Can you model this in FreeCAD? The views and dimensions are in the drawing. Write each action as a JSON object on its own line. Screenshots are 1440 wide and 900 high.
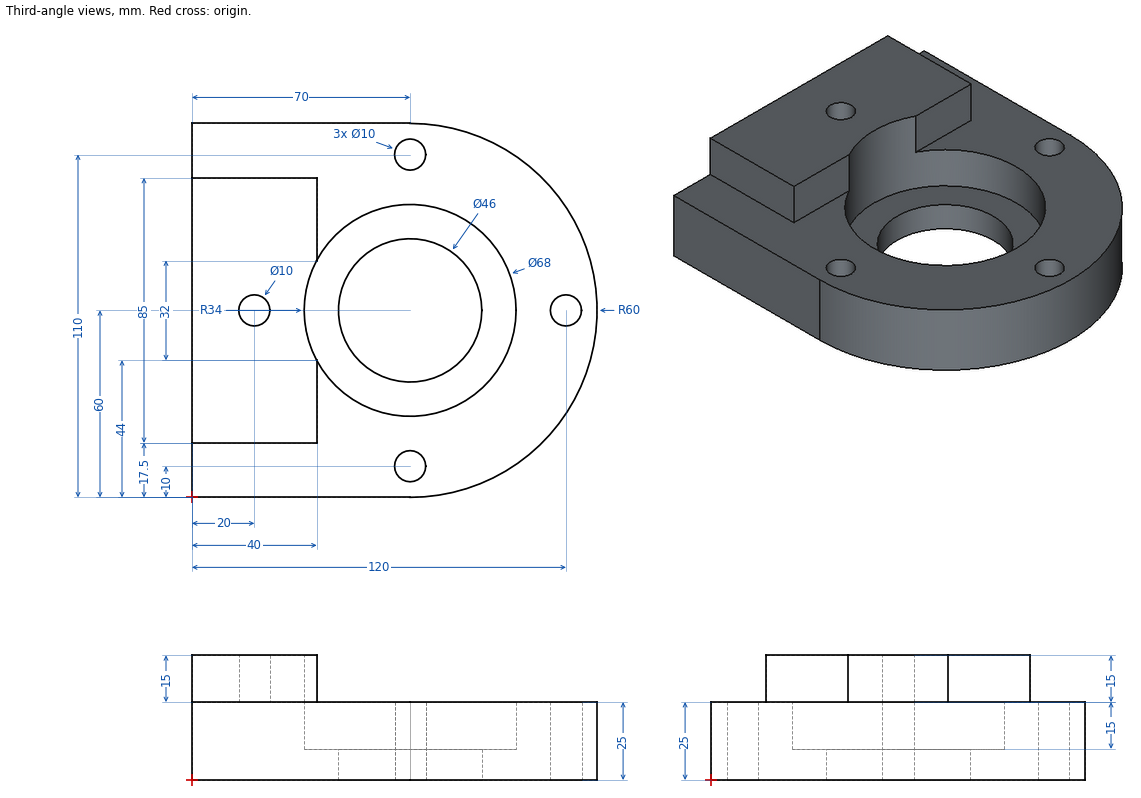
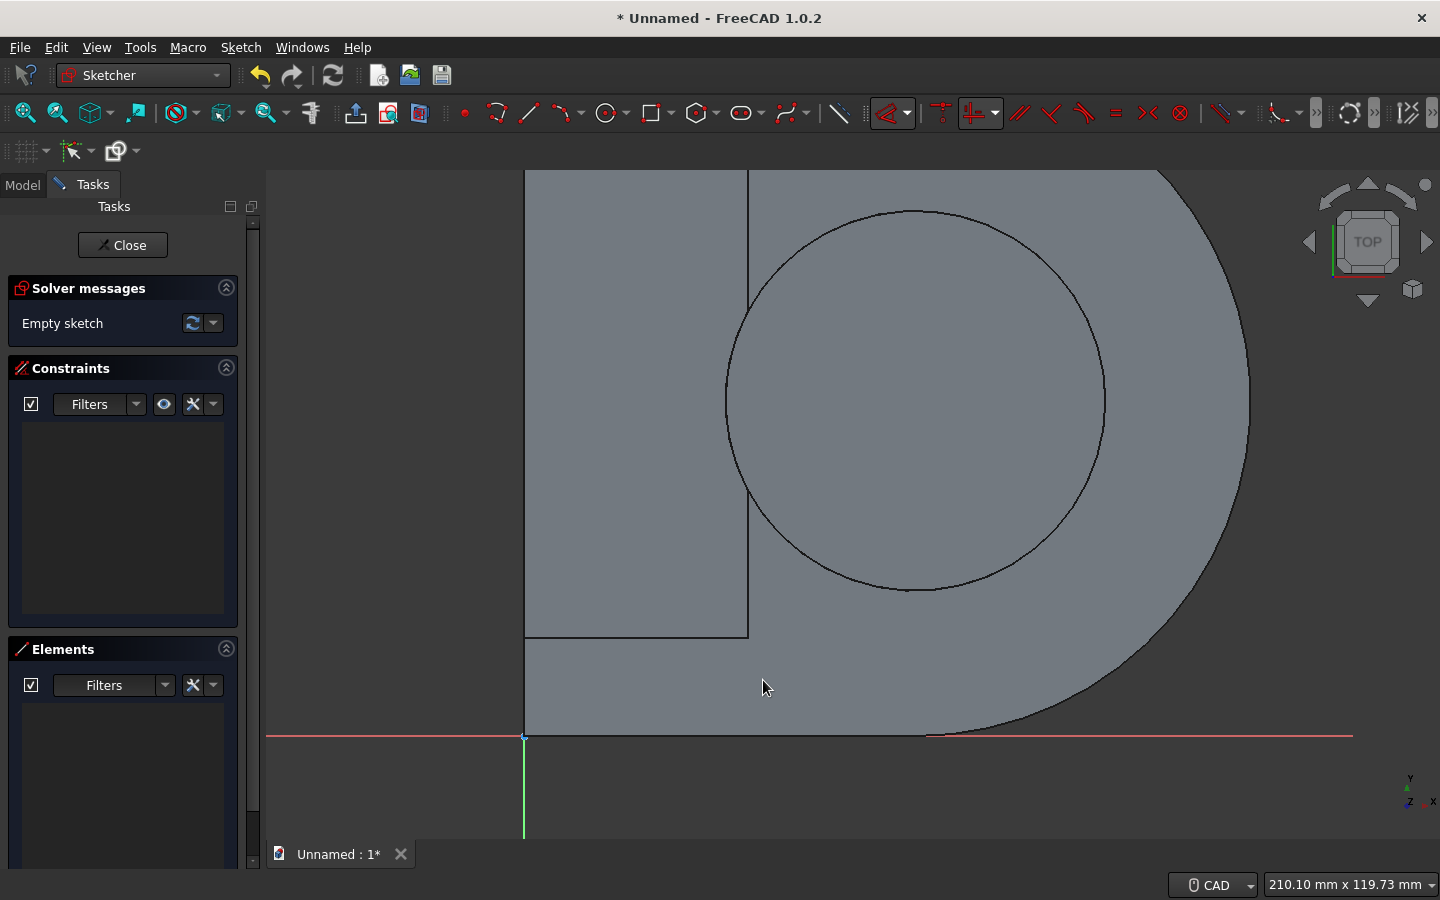
{"action": "left_click", "coordinate": [606, 114]}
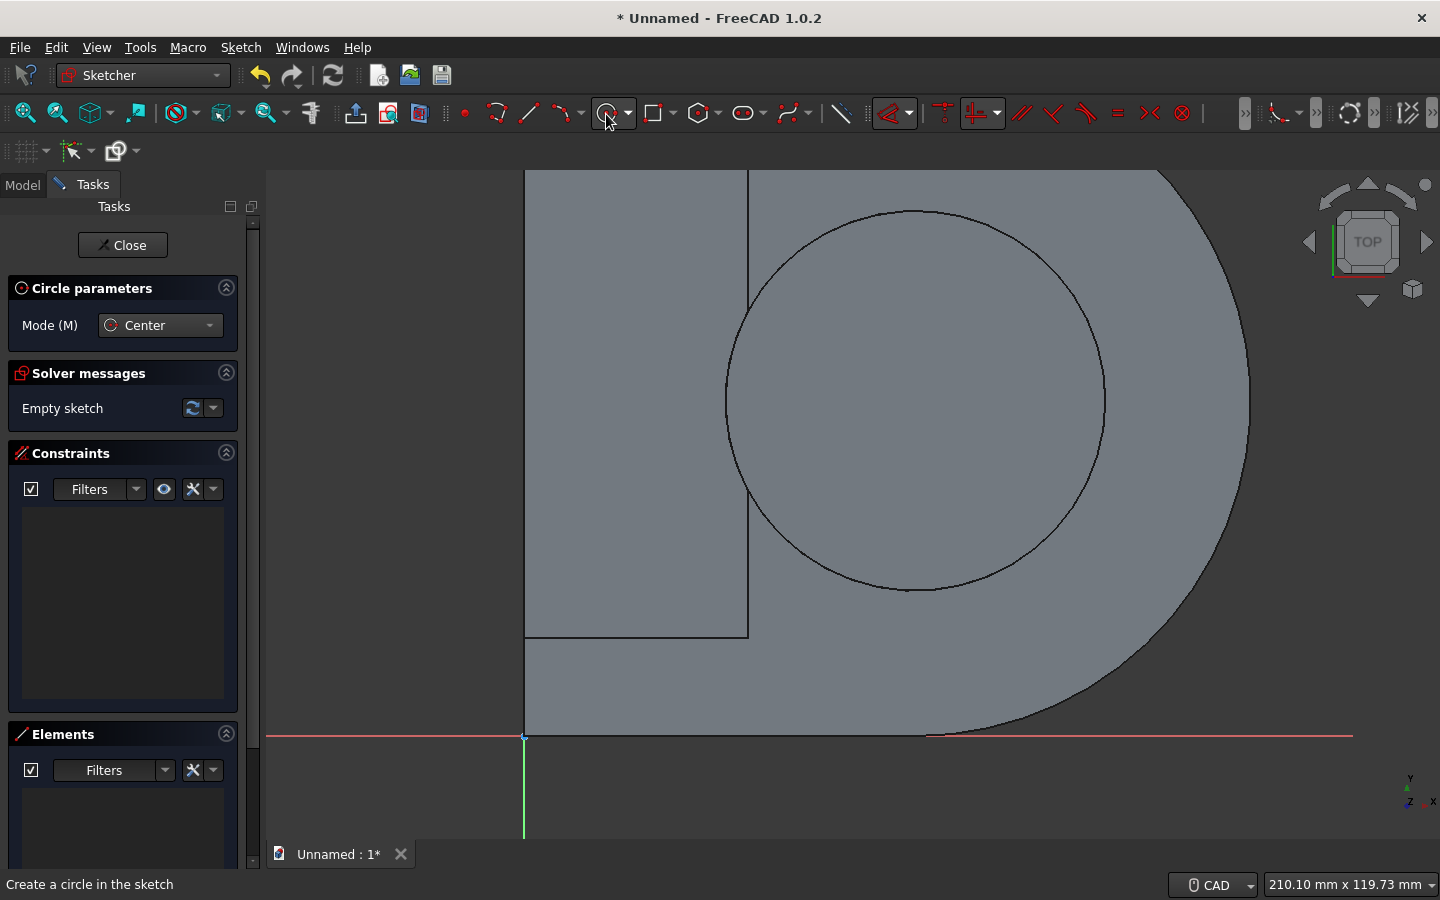
{"action": "left_click", "coordinate": [915, 401]}
{"action": "left_click", "coordinate": [1006, 310]}
{"action": "key", "text": "Escape"}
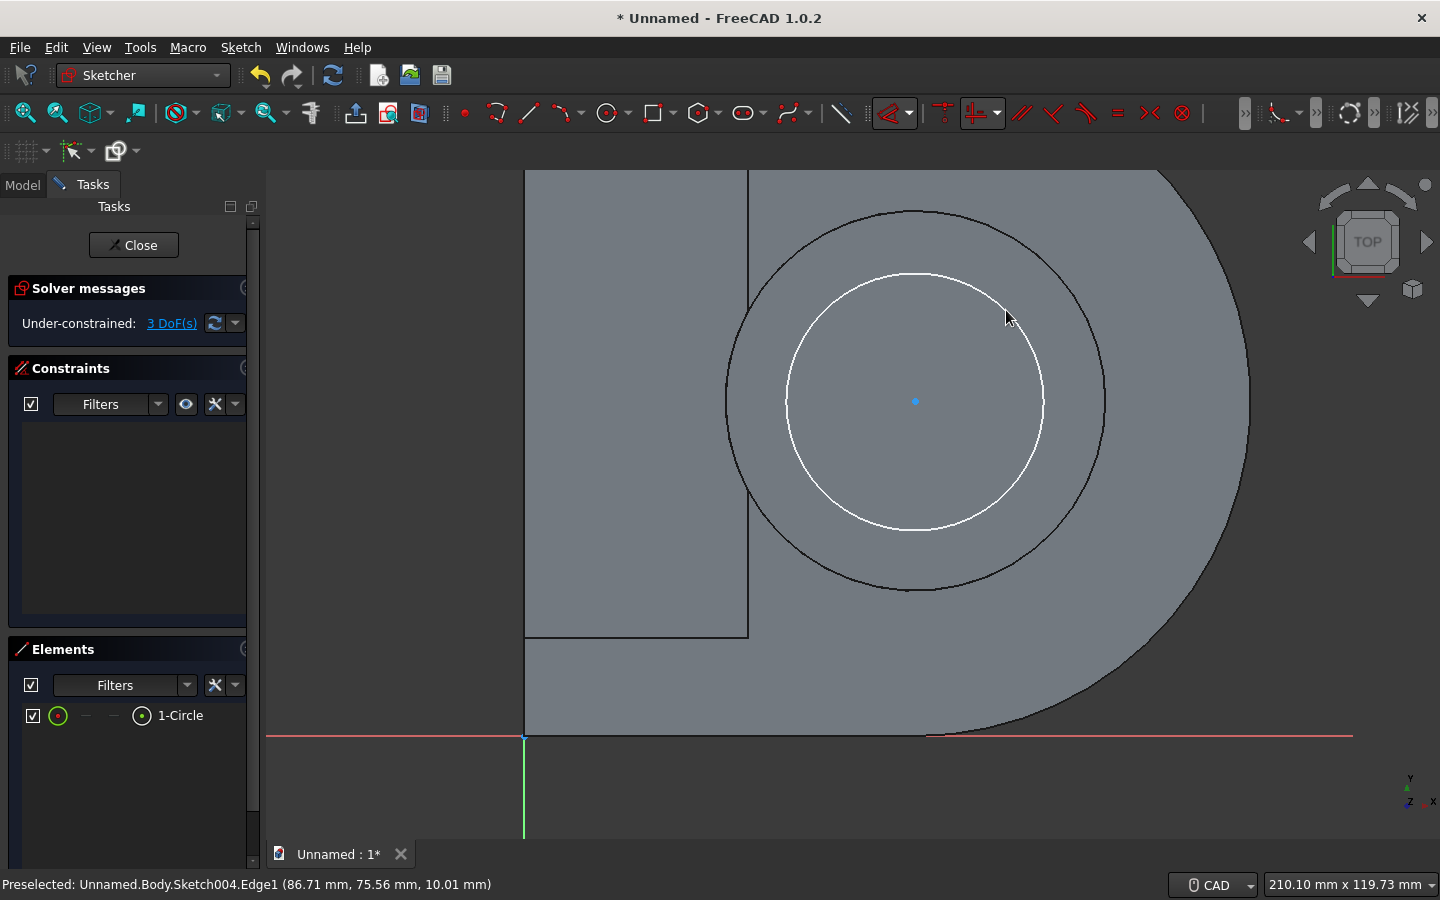
{"action": "left_click", "coordinate": [1006, 311]}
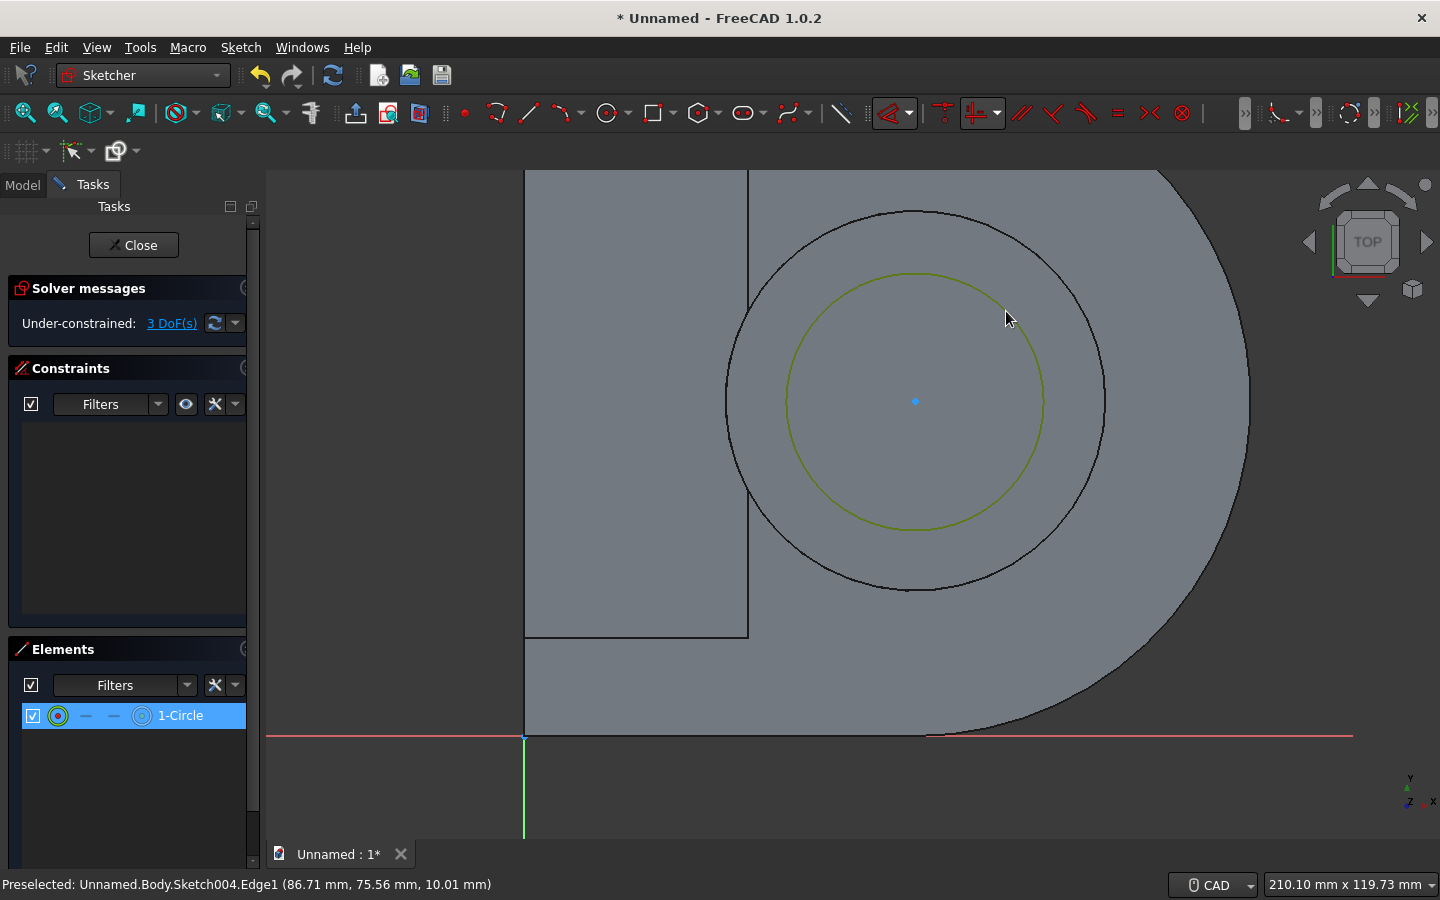
{"action": "left_click", "coordinate": [912, 114]}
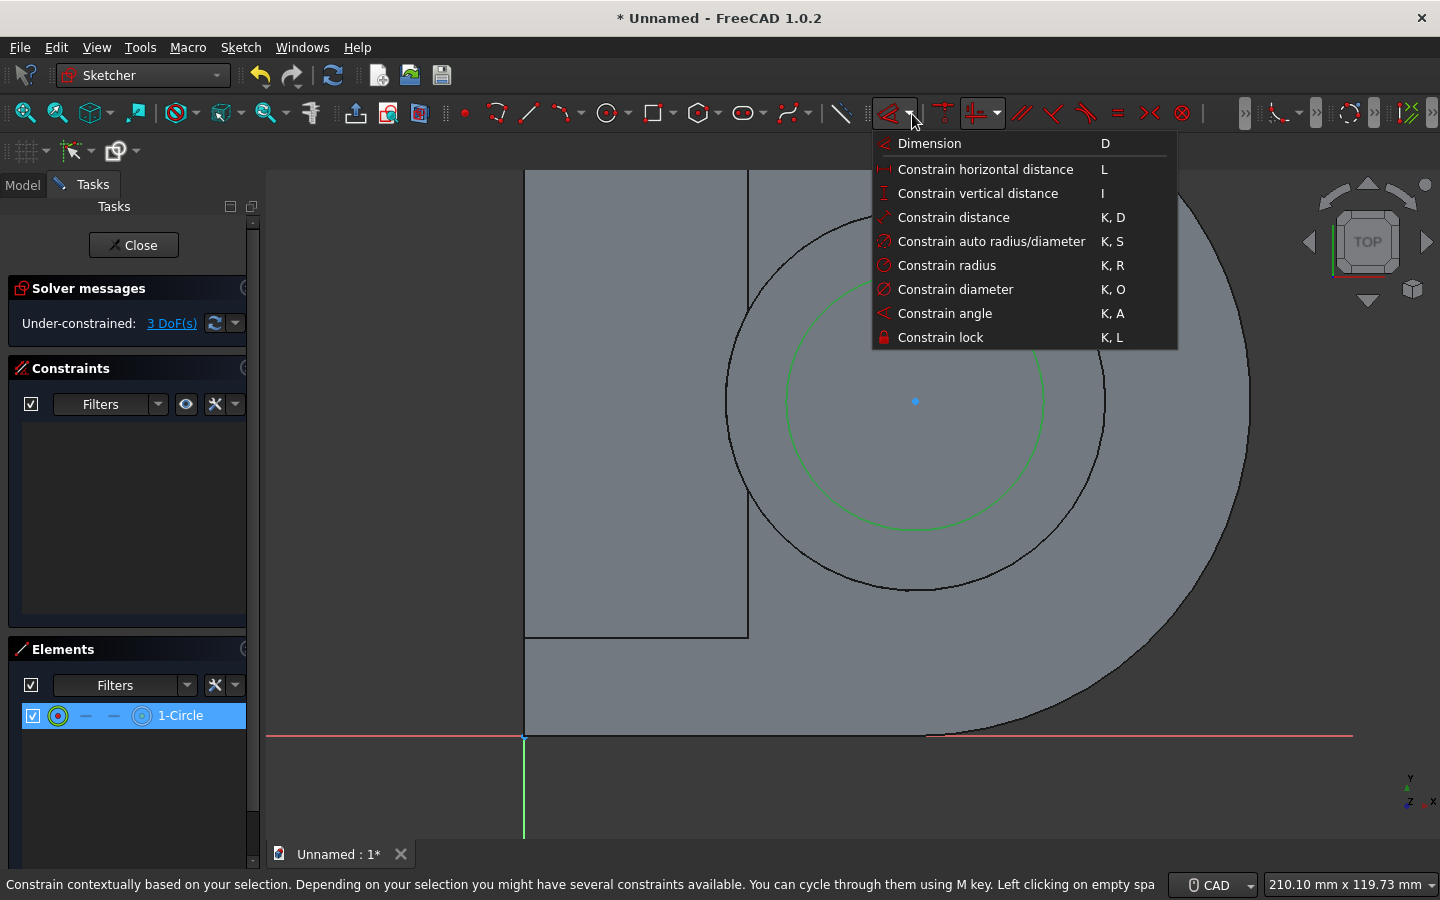
{"action": "left_click", "coordinate": [1025, 289]}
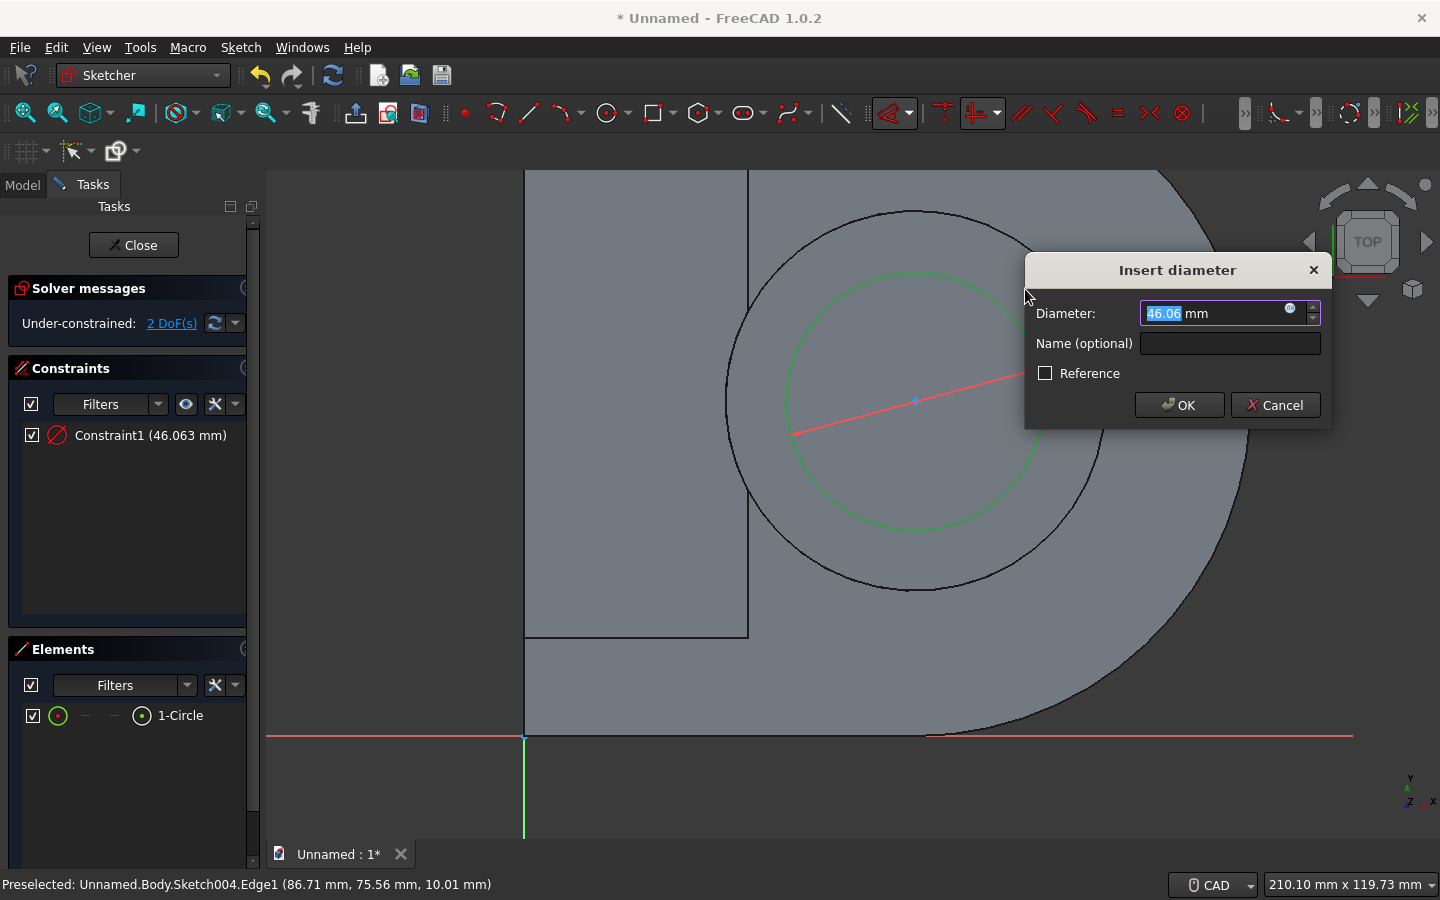
{"action": "type", "text": "46"}
{"action": "key", "text": "Return"}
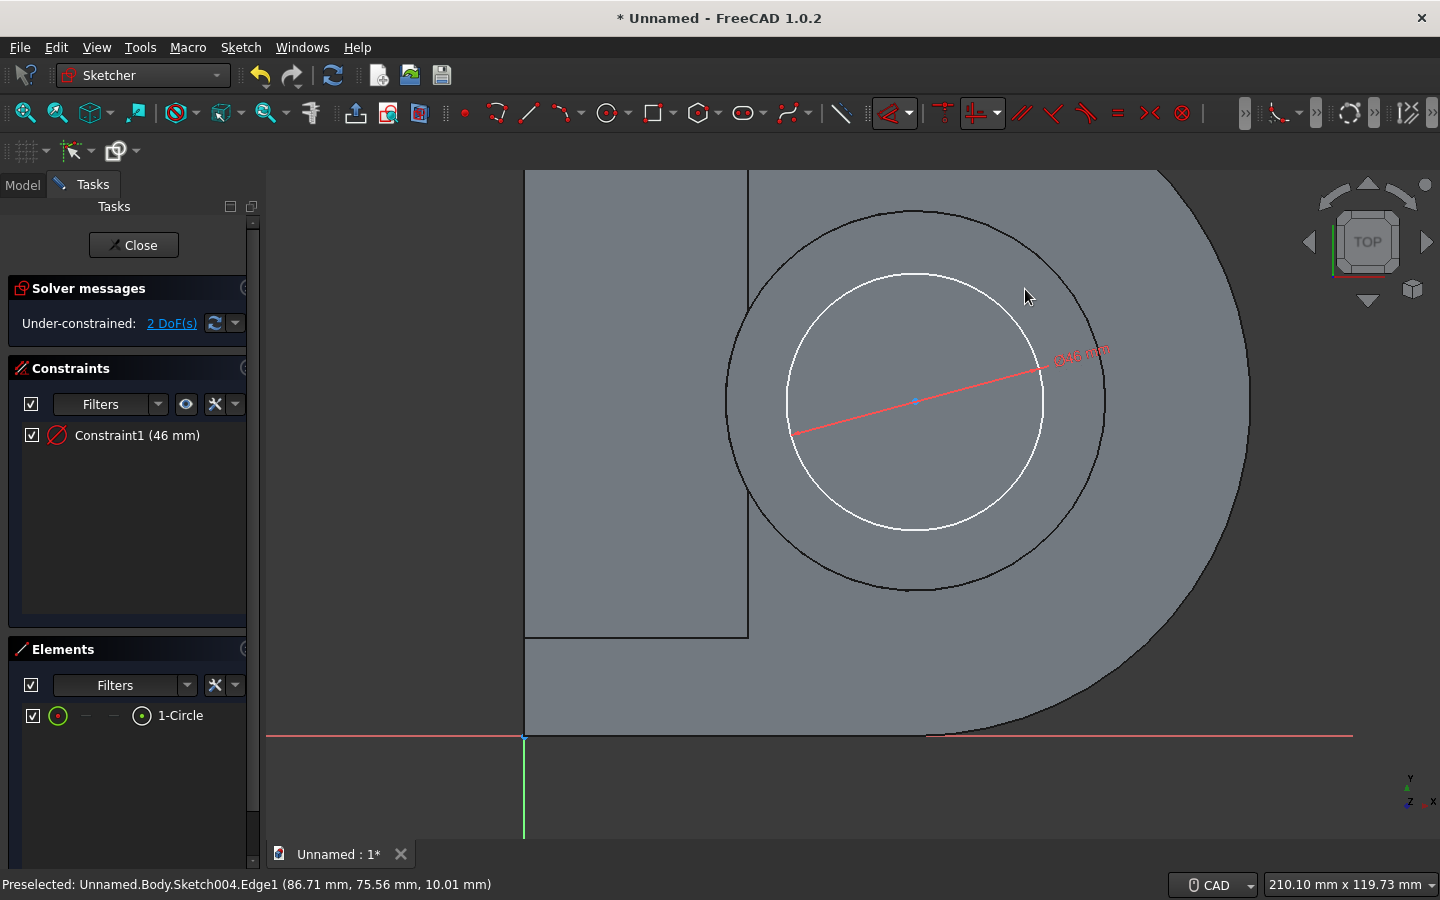
{"action": "left_click", "coordinate": [915, 402]}